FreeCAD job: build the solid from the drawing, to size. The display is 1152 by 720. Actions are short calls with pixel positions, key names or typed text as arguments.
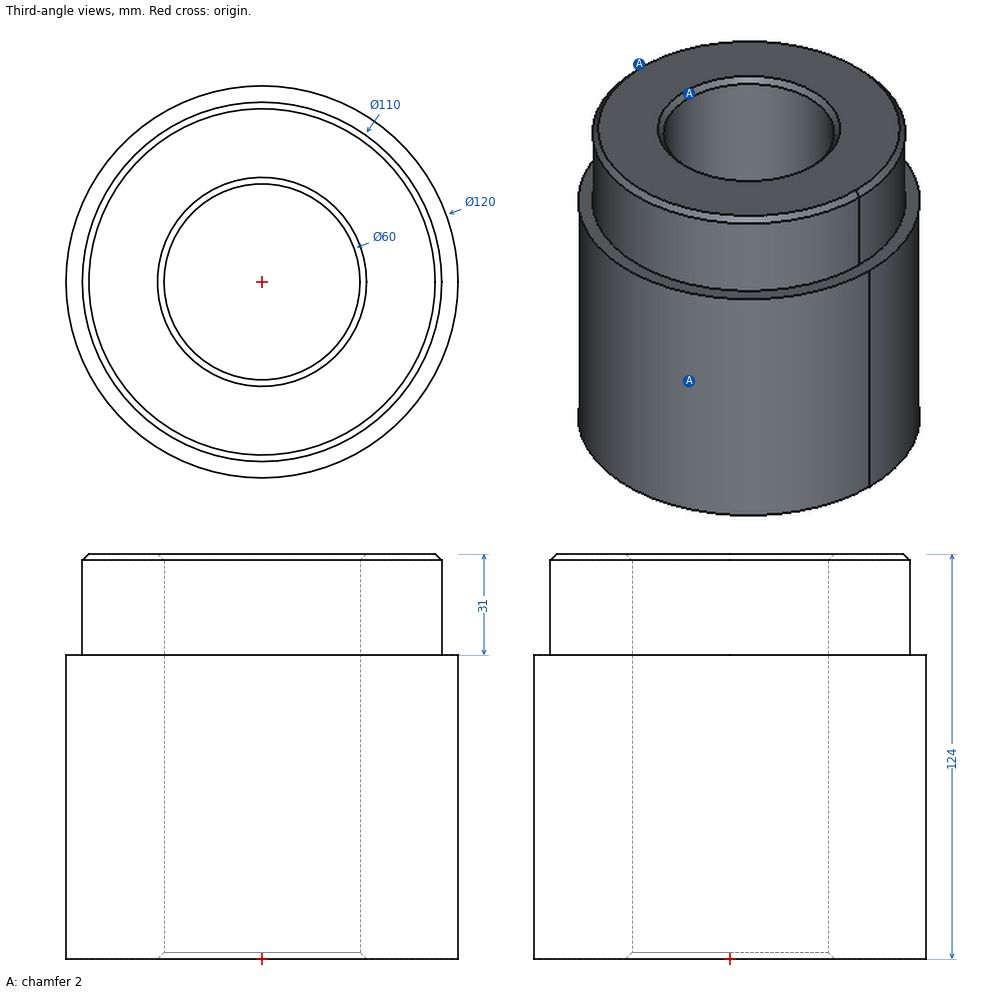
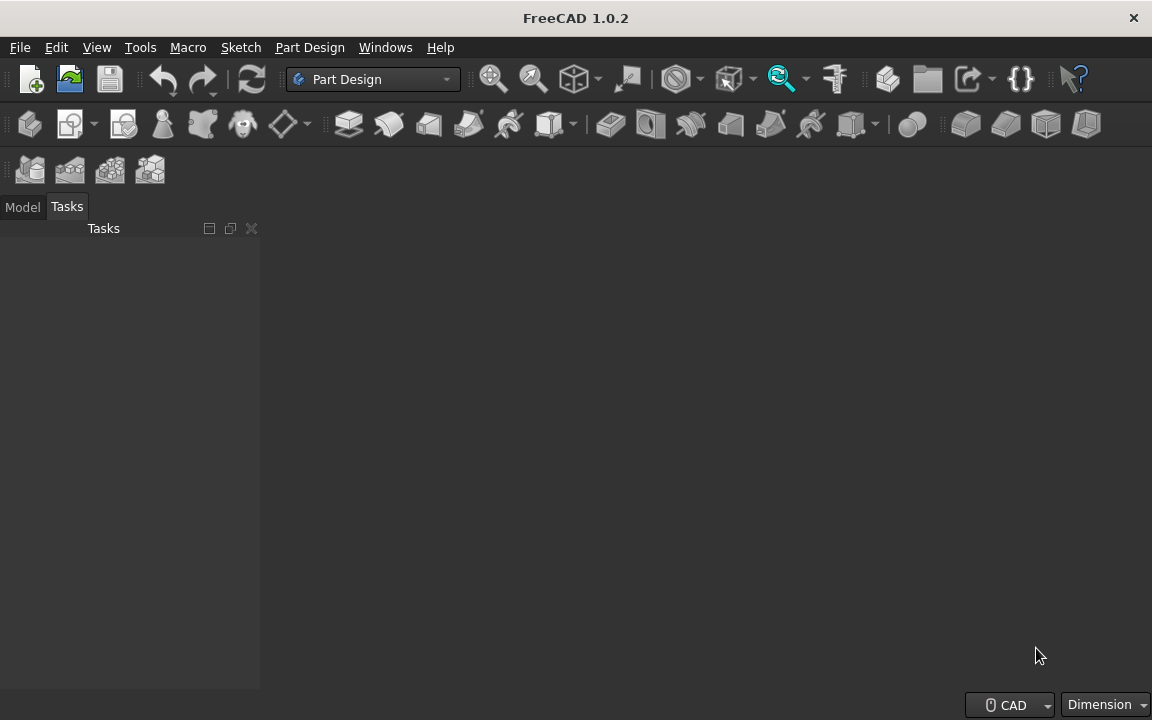
key(ctrl+n)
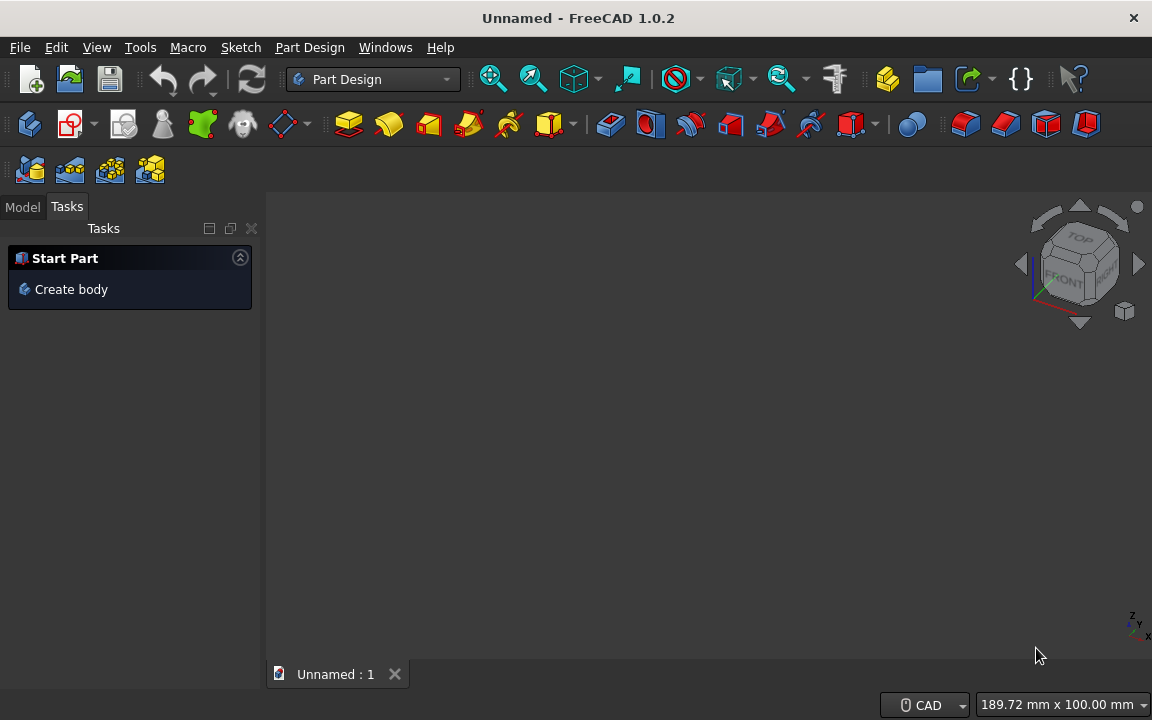
click(70, 124)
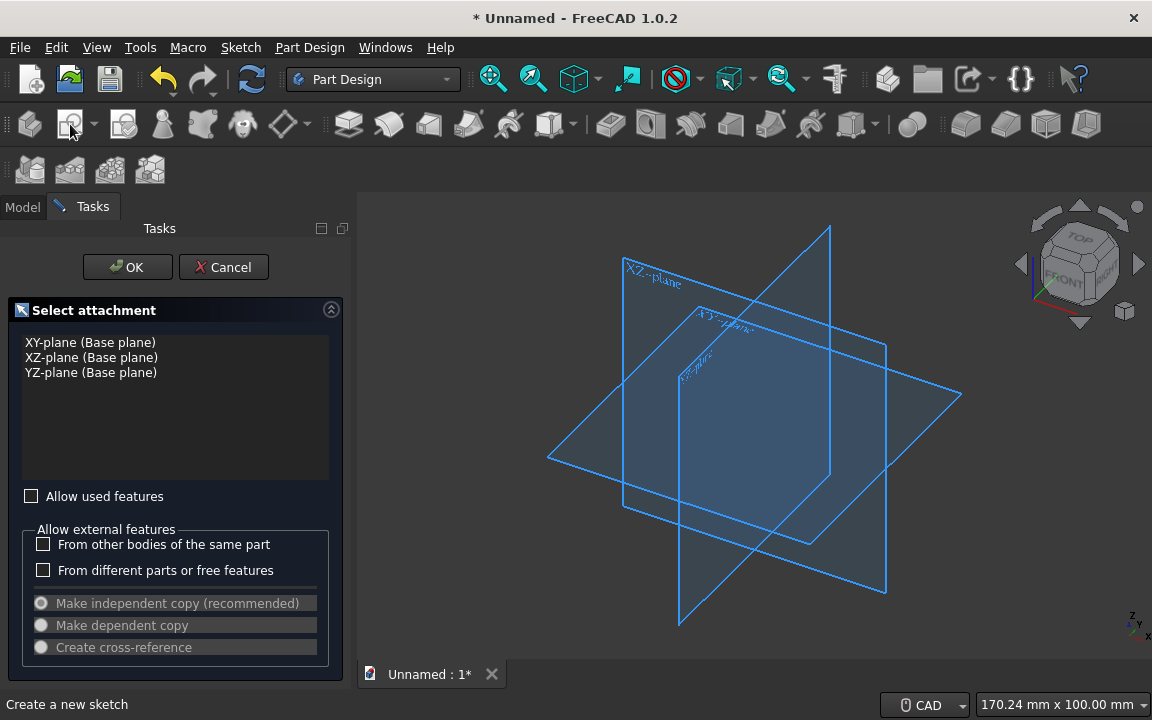
click(82, 342)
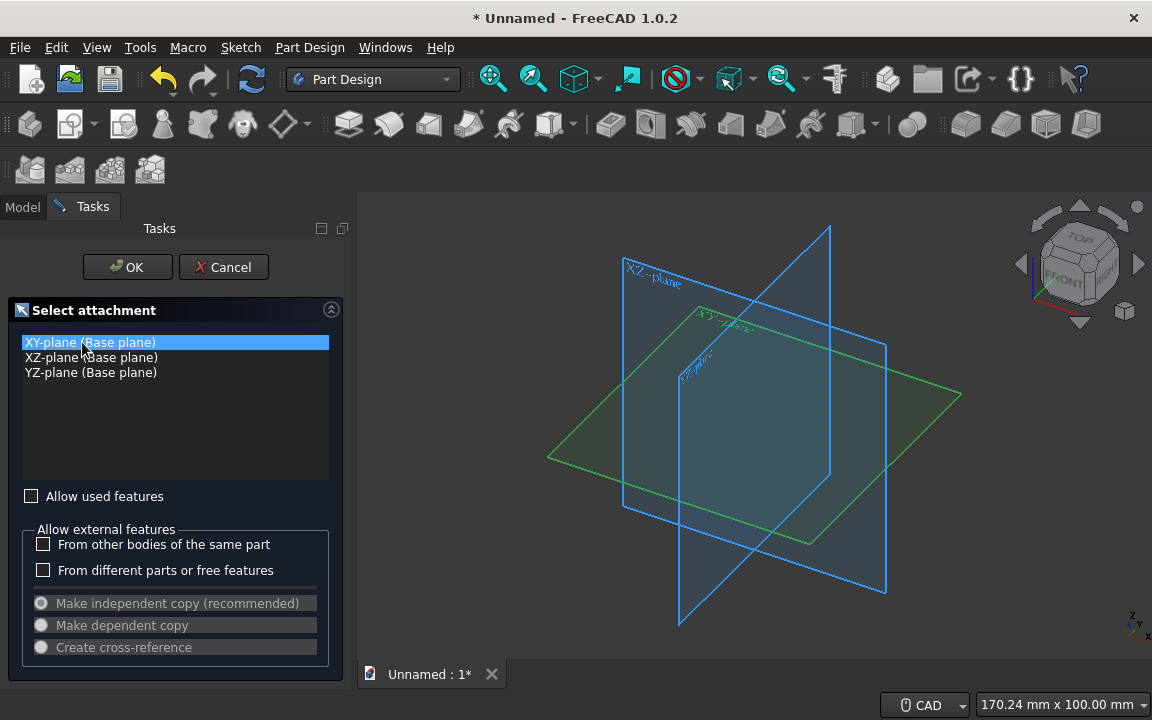
click(128, 267)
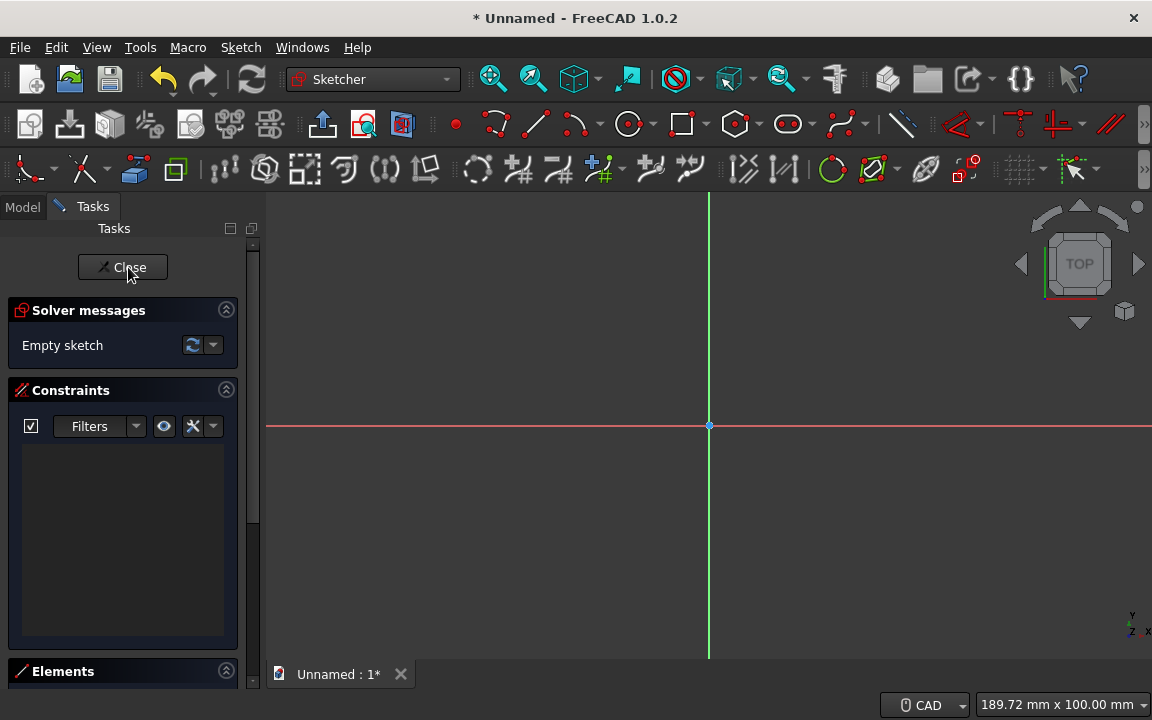
scroll(557, 426, down, 3)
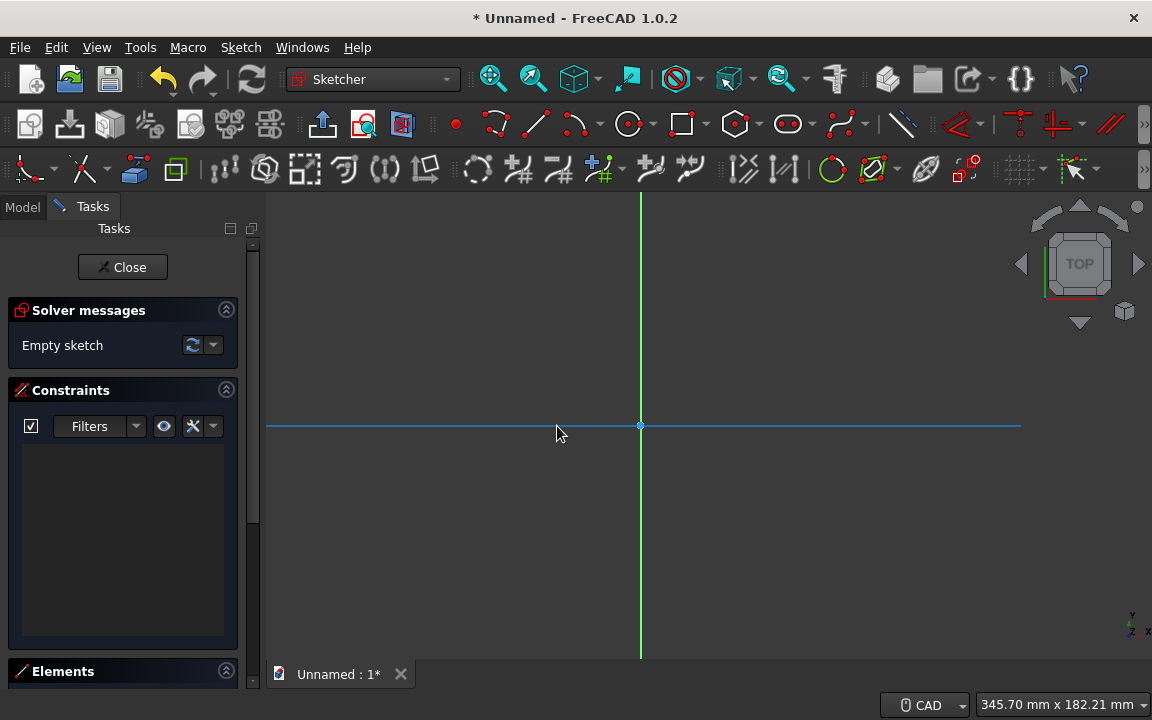
click(630, 124)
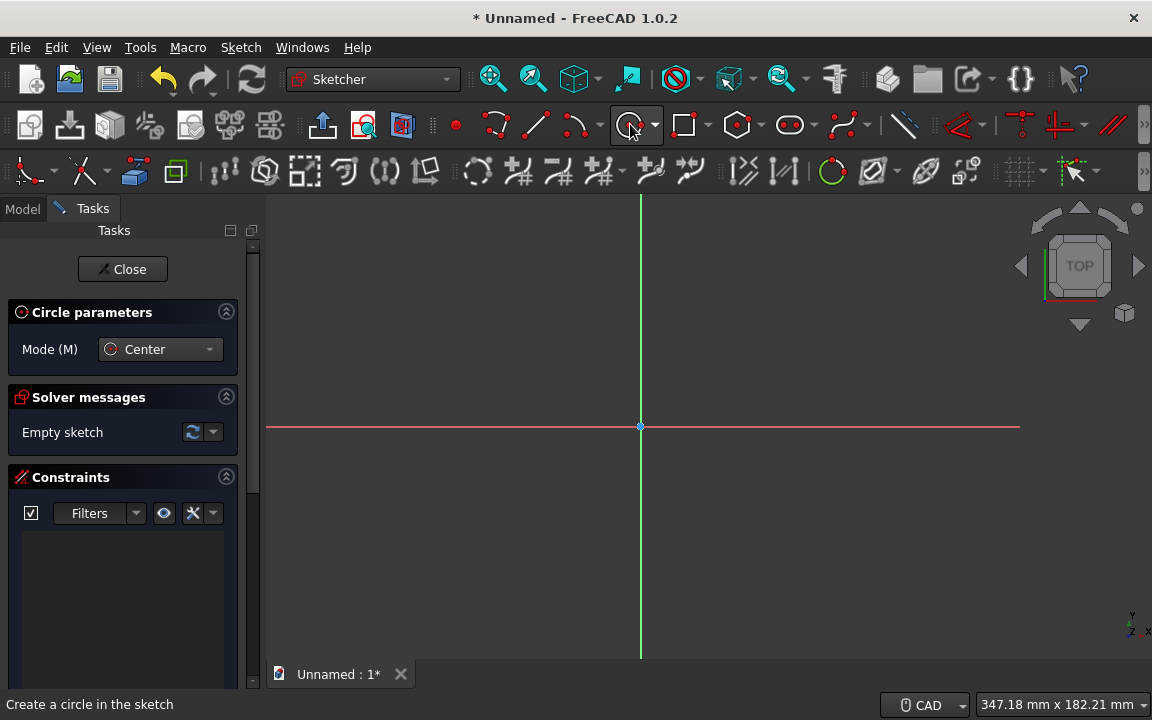
click(641, 427)
click(749, 319)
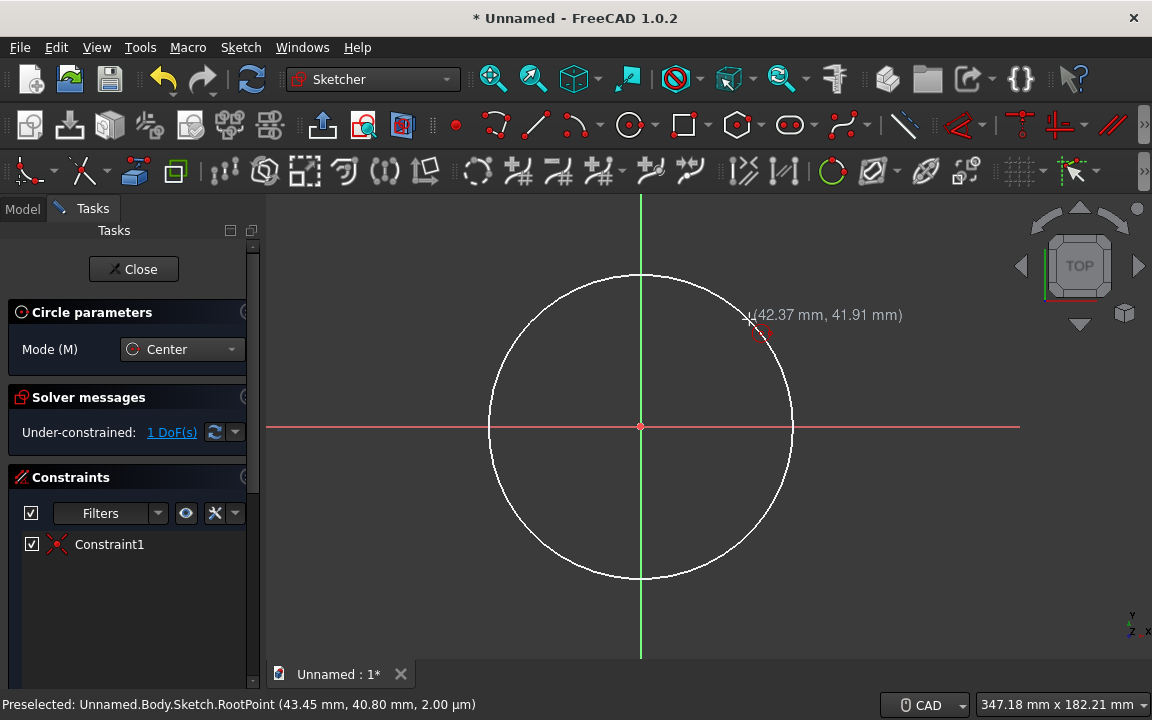
click(641, 427)
click(695, 373)
key(Escape)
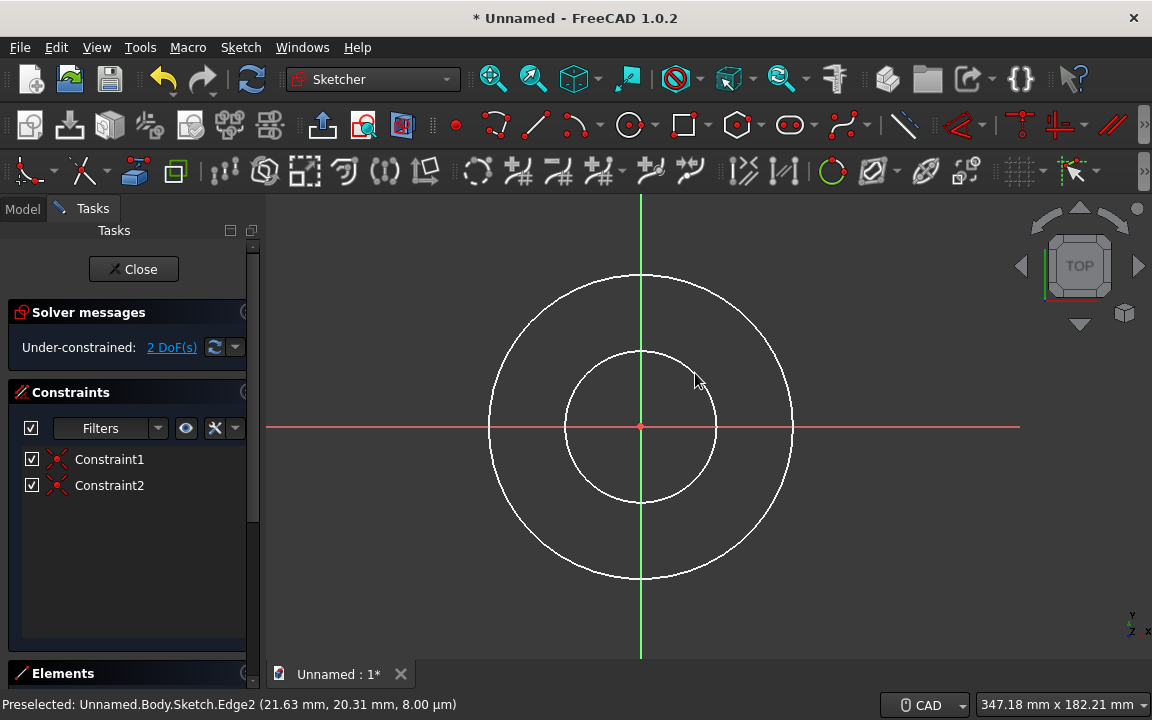
click(958, 126)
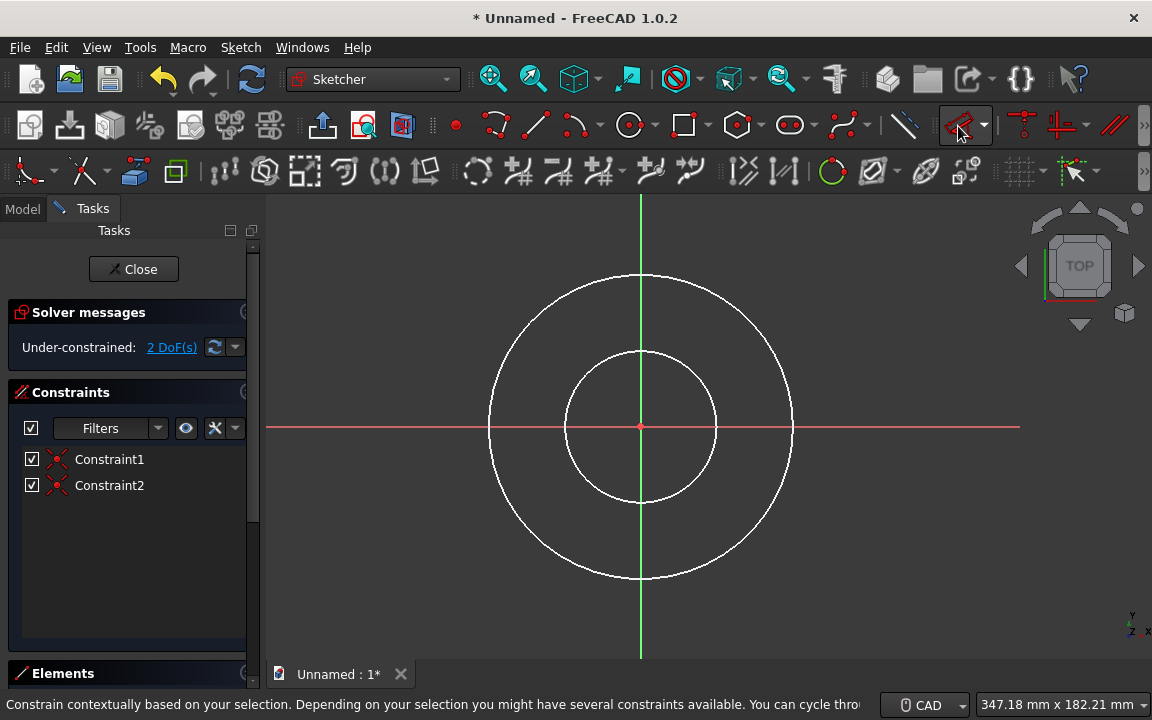
click(748, 319)
click(771, 296)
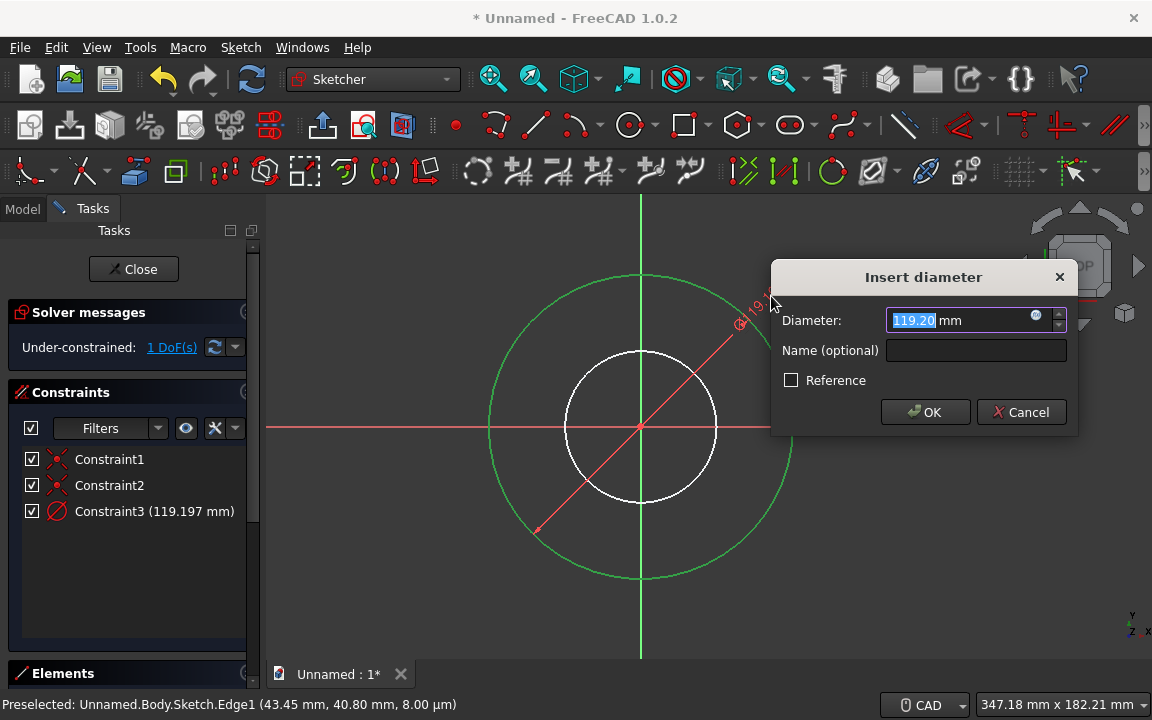
text(120)
key(Return)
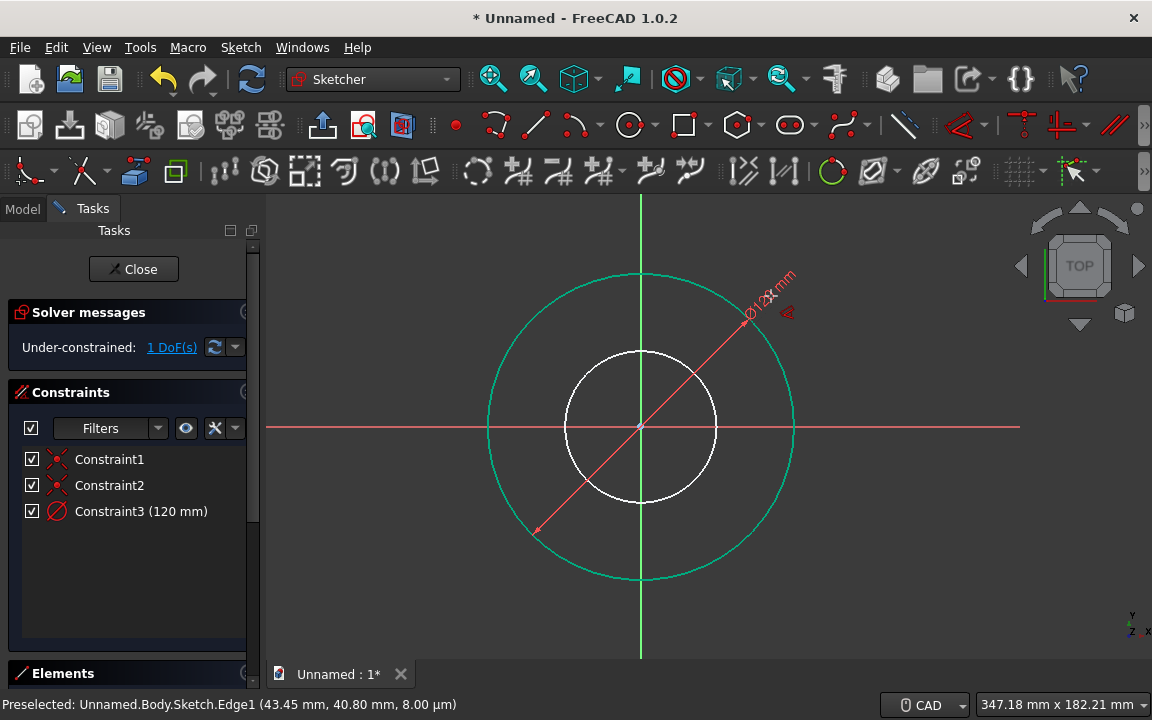
click(694, 373)
click(716, 350)